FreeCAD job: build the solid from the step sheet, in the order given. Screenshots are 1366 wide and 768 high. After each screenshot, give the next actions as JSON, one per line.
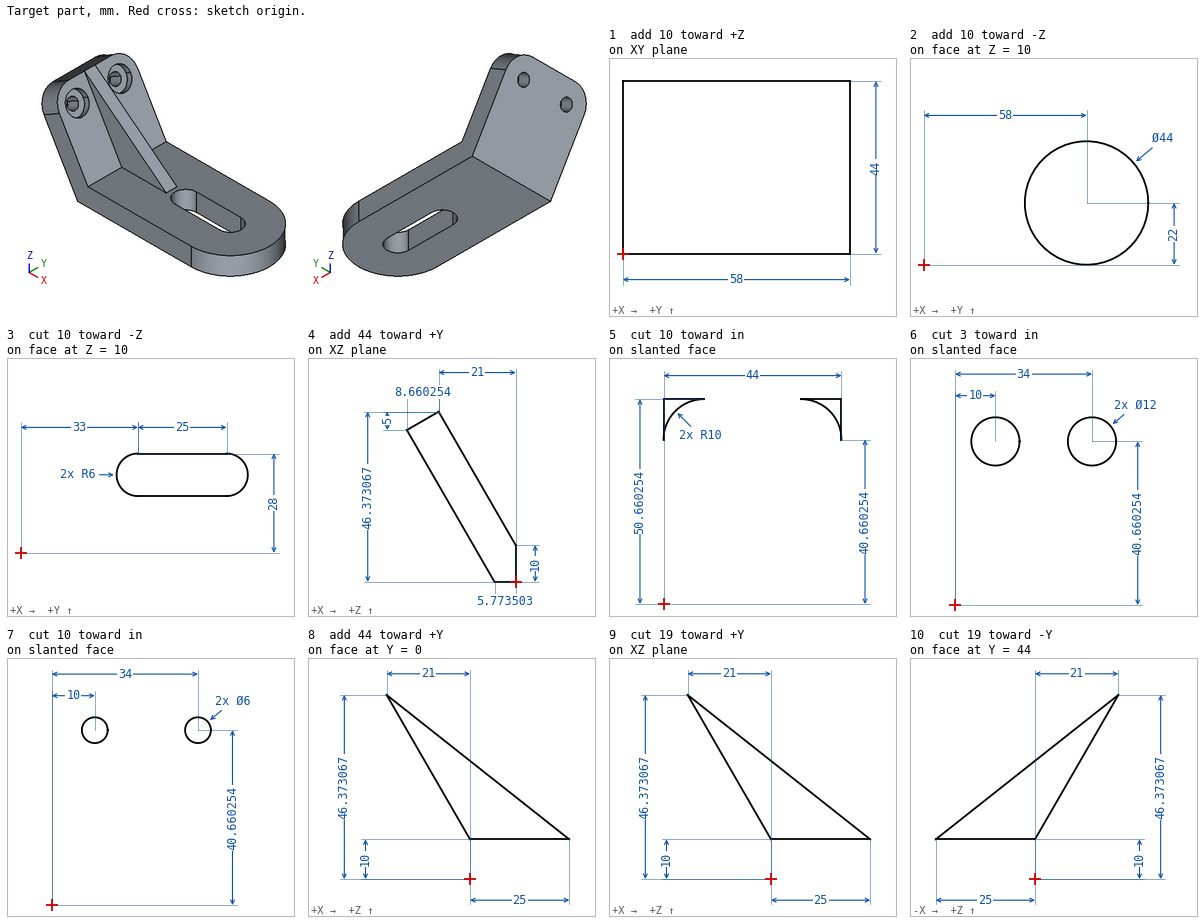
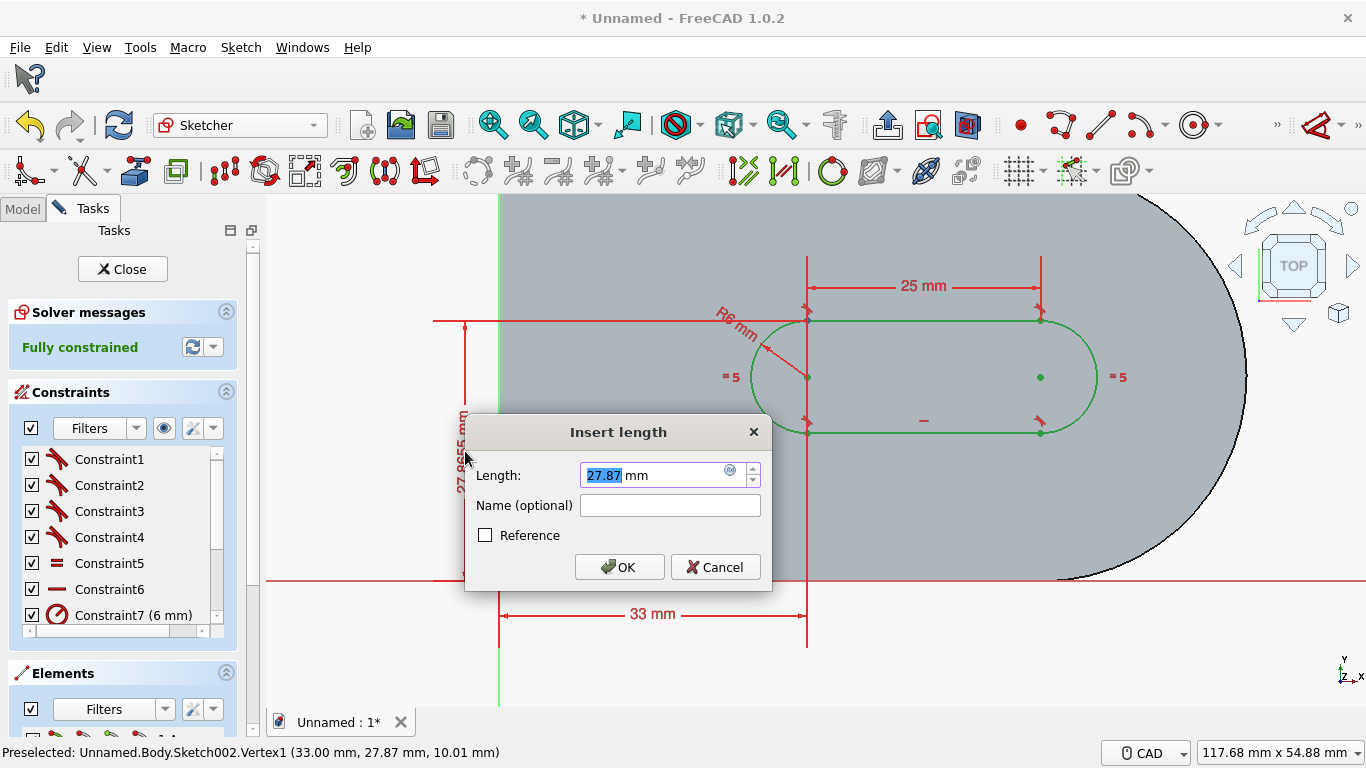
{"action": "type", "text": "28"}
{"action": "key", "text": "Return"}
{"action": "key", "text": "Escape"}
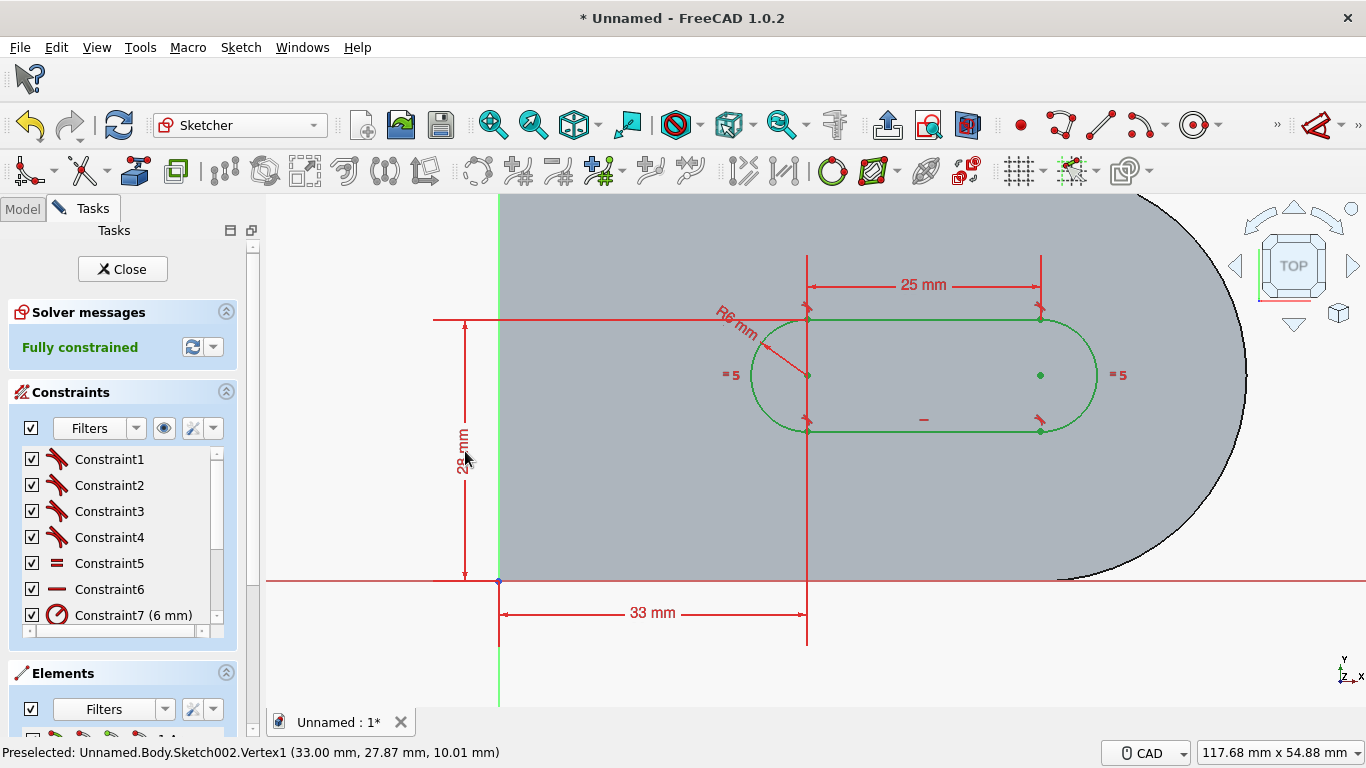
{"action": "left_click", "coordinate": [123, 269]}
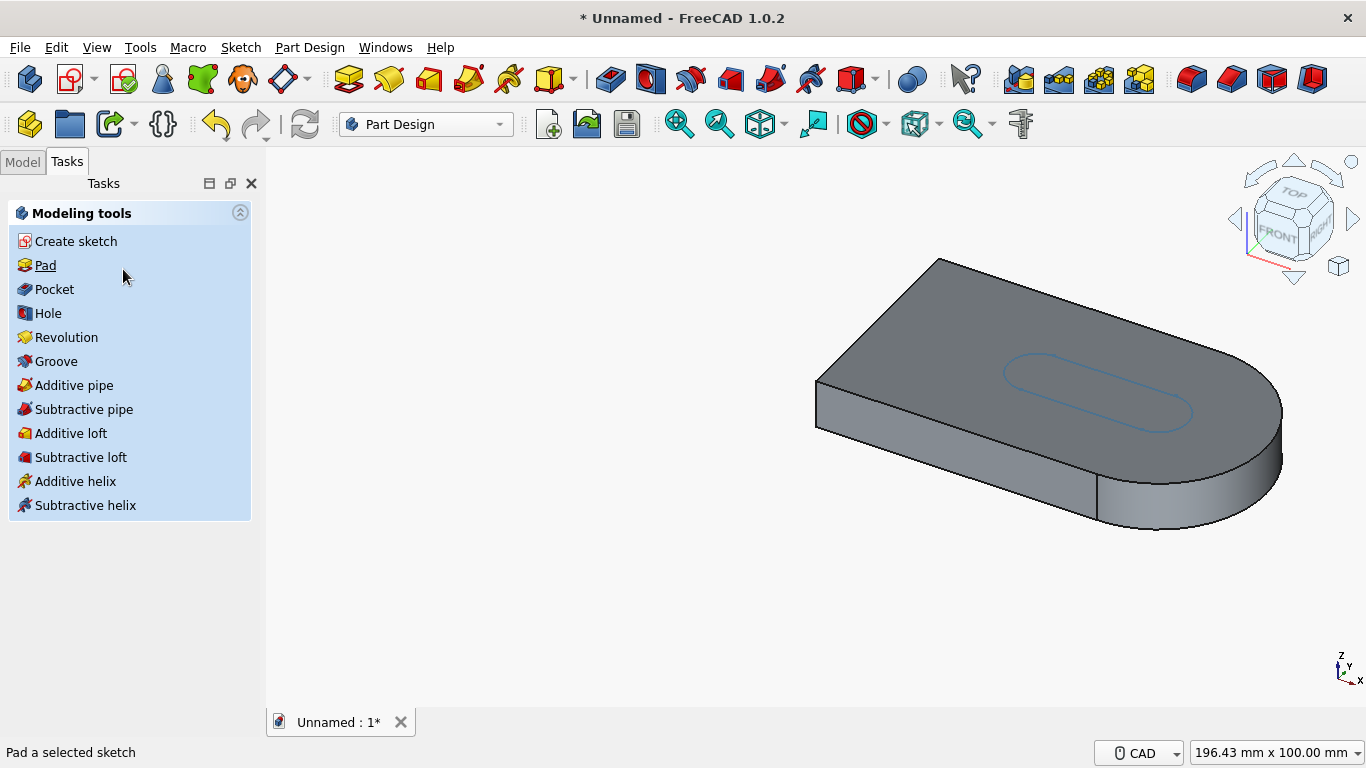
{"action": "left_click", "coordinate": [612, 80]}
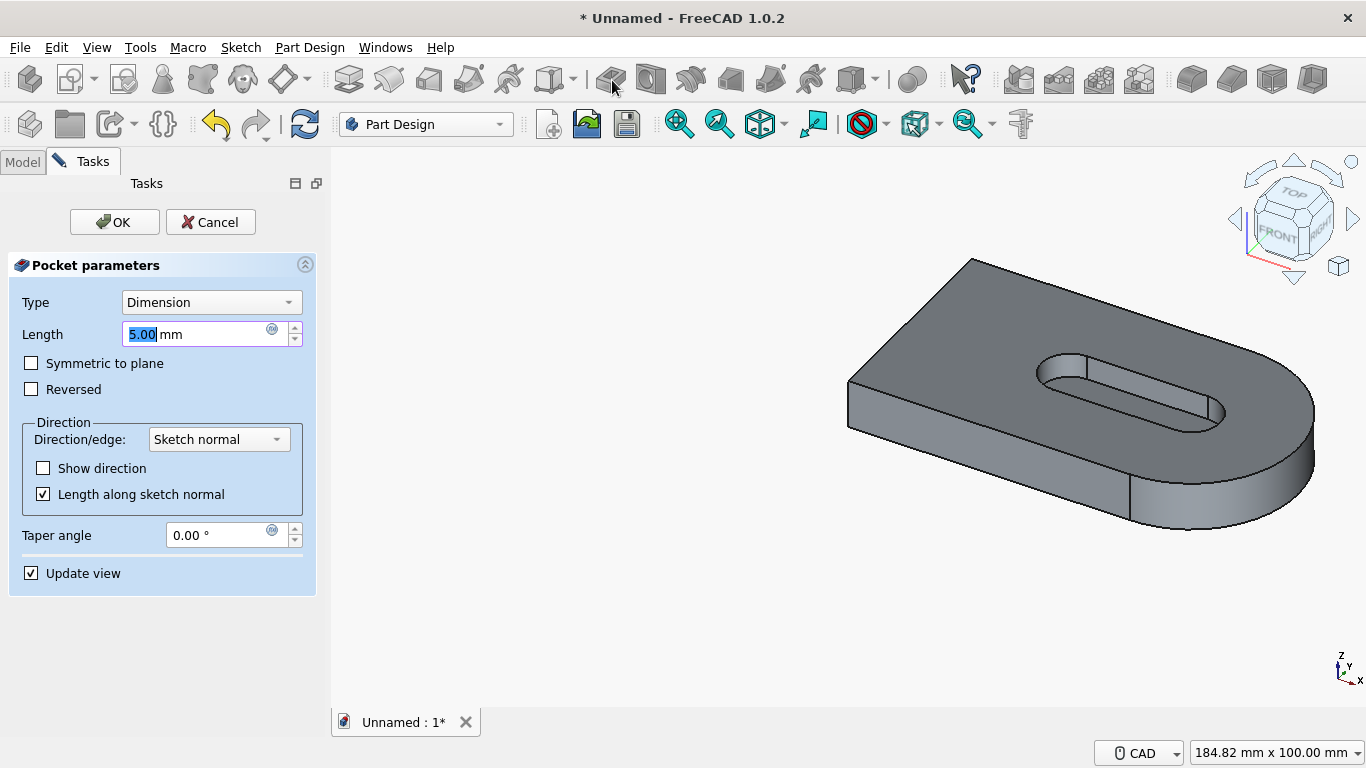
{"action": "type", "text": "10"}
{"action": "key", "text": "Tab"}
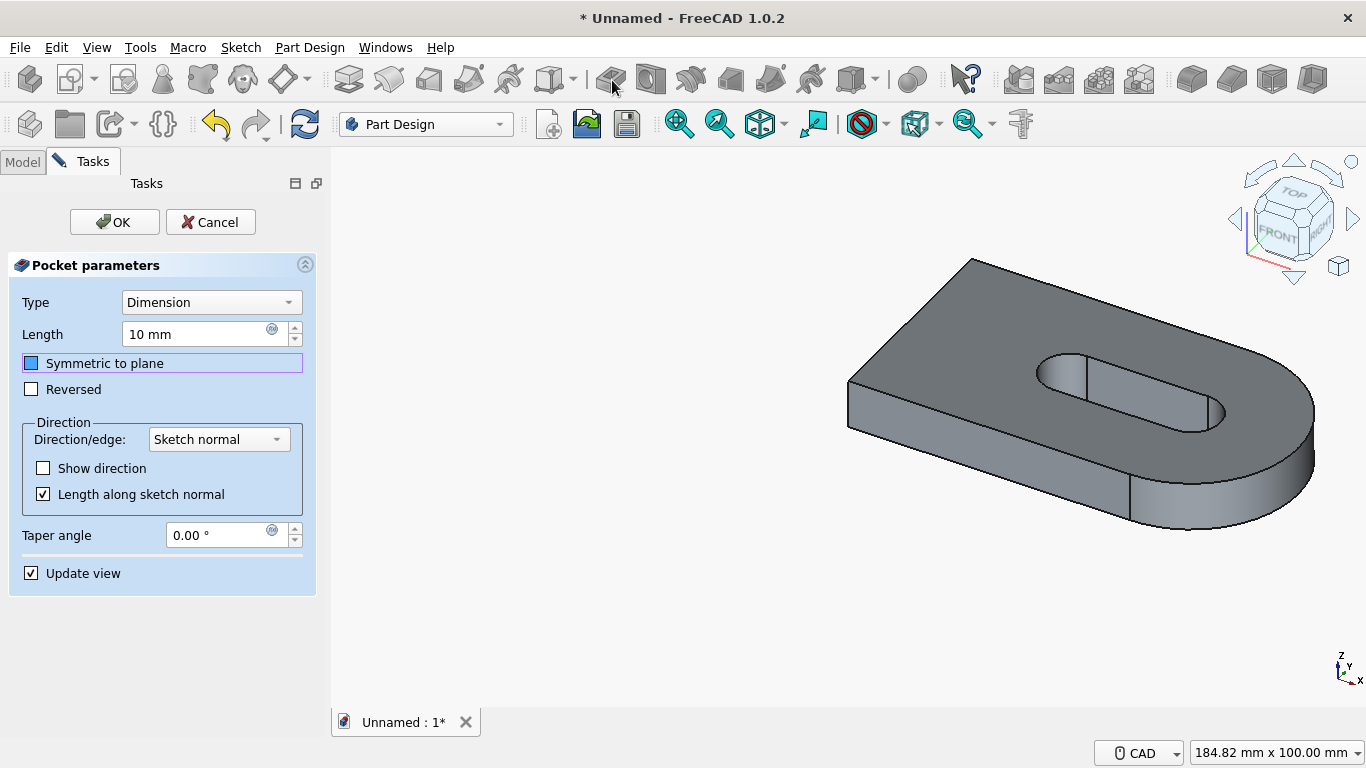
{"action": "left_click", "coordinate": [115, 222]}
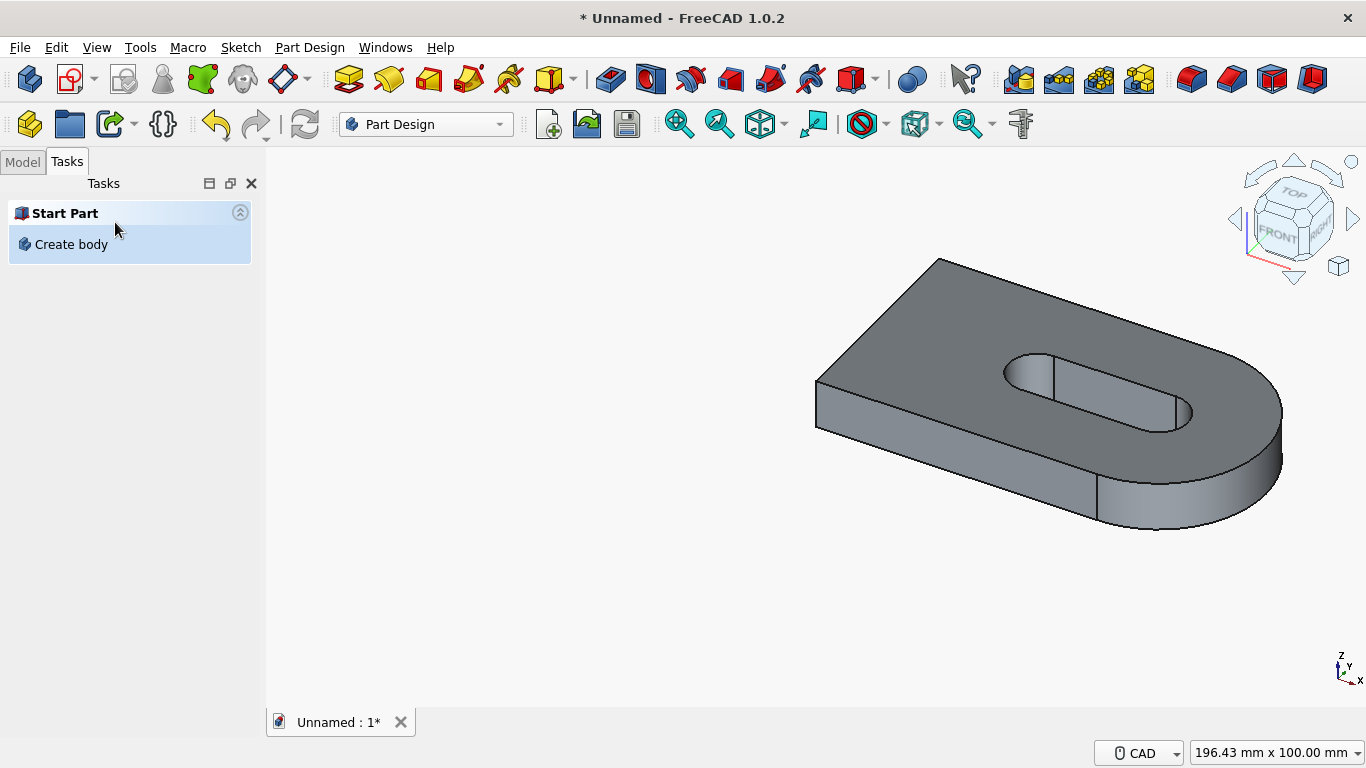
{"action": "left_click", "coordinate": [70, 80]}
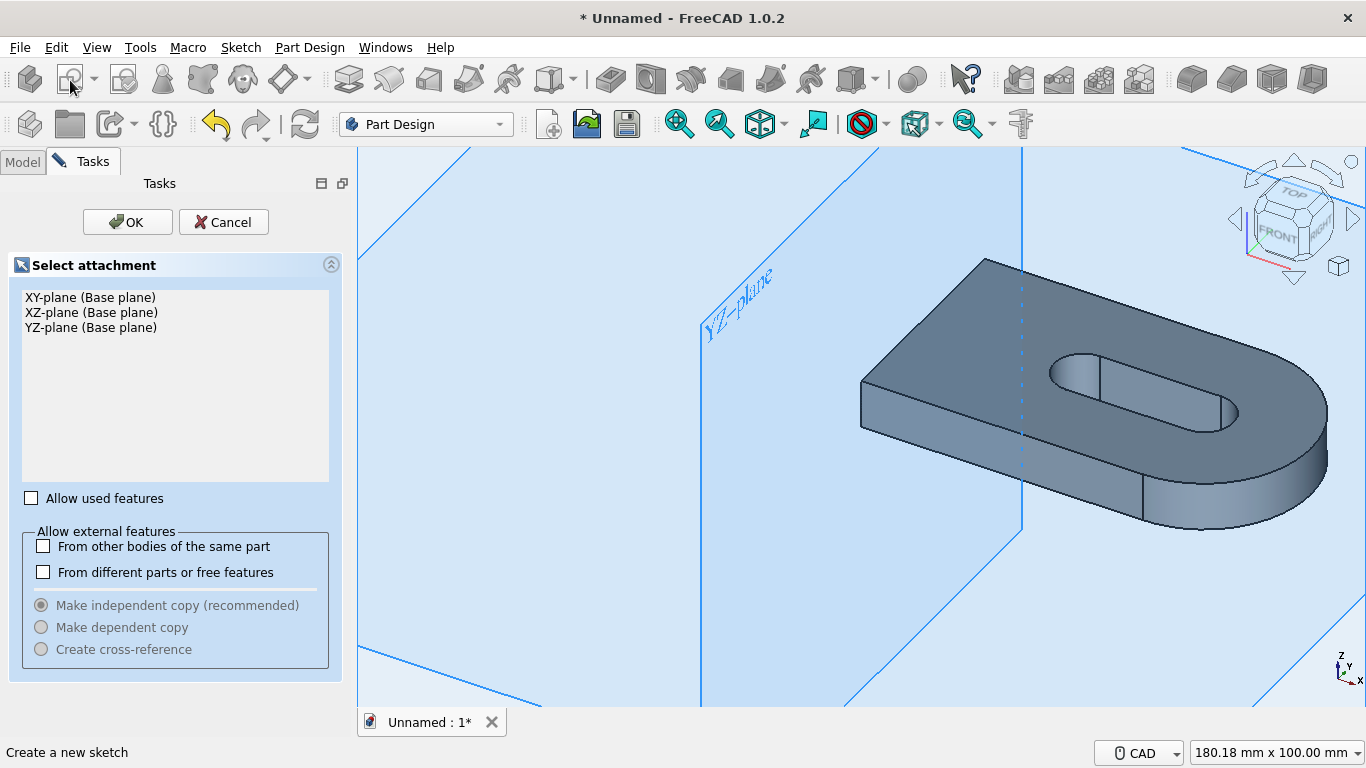
{"action": "left_click", "coordinate": [82, 312]}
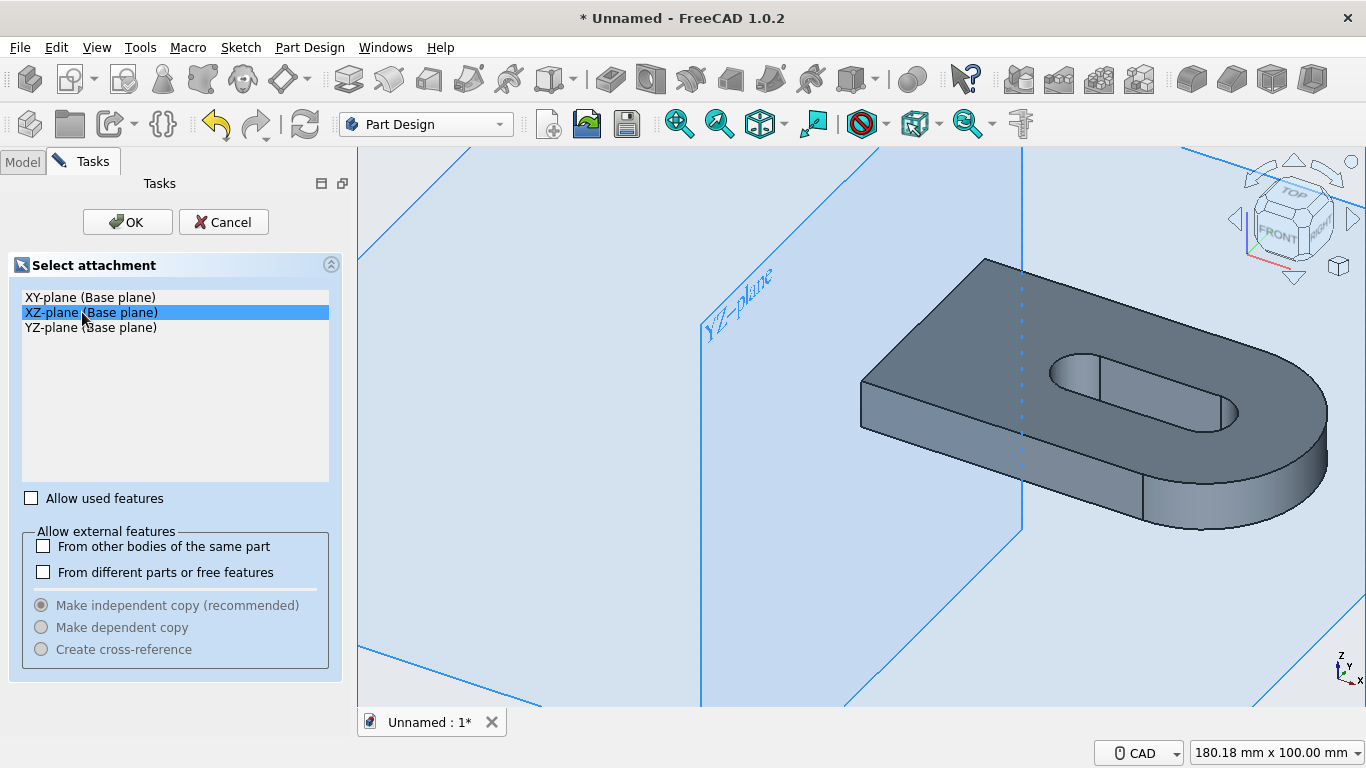
{"action": "left_click", "coordinate": [128, 222]}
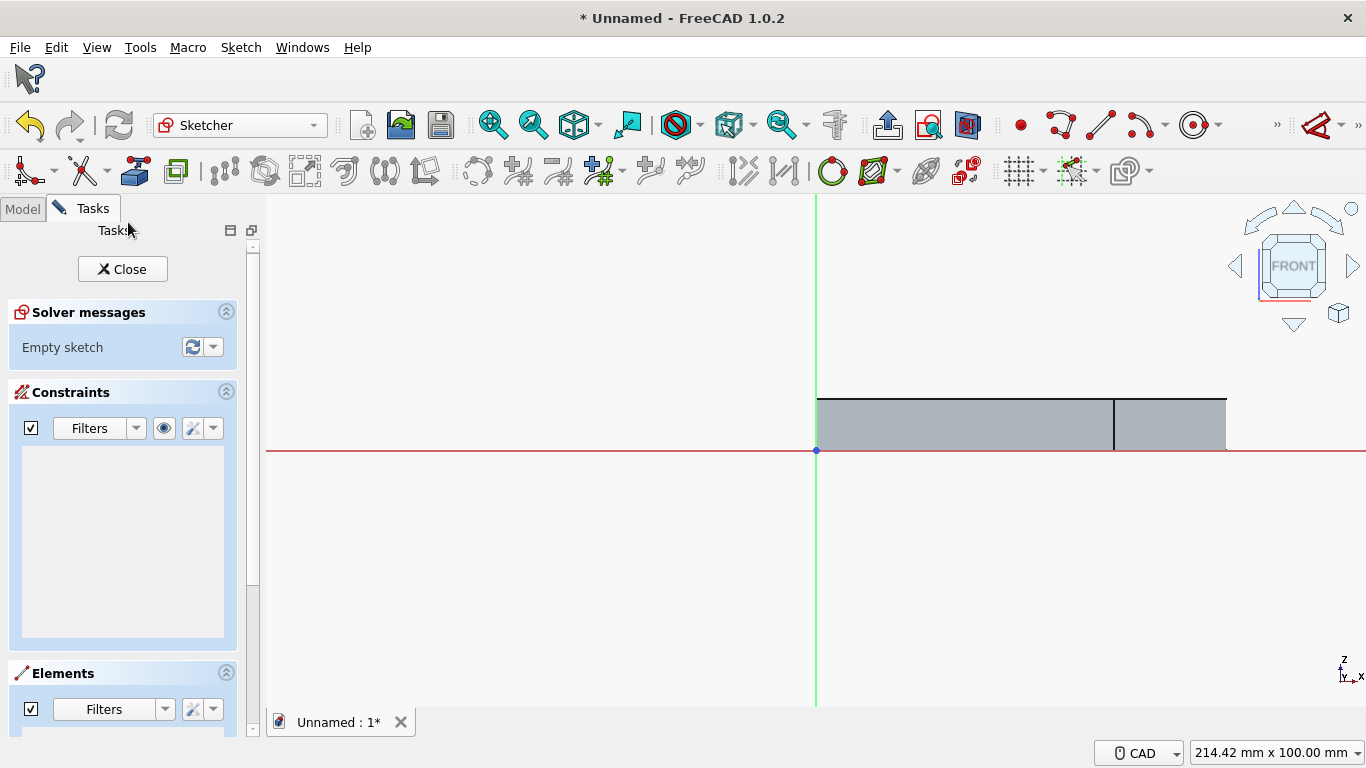
{"action": "scroll", "coordinate": [782, 679], "scroll_direction": "down", "scroll_amount": 1}